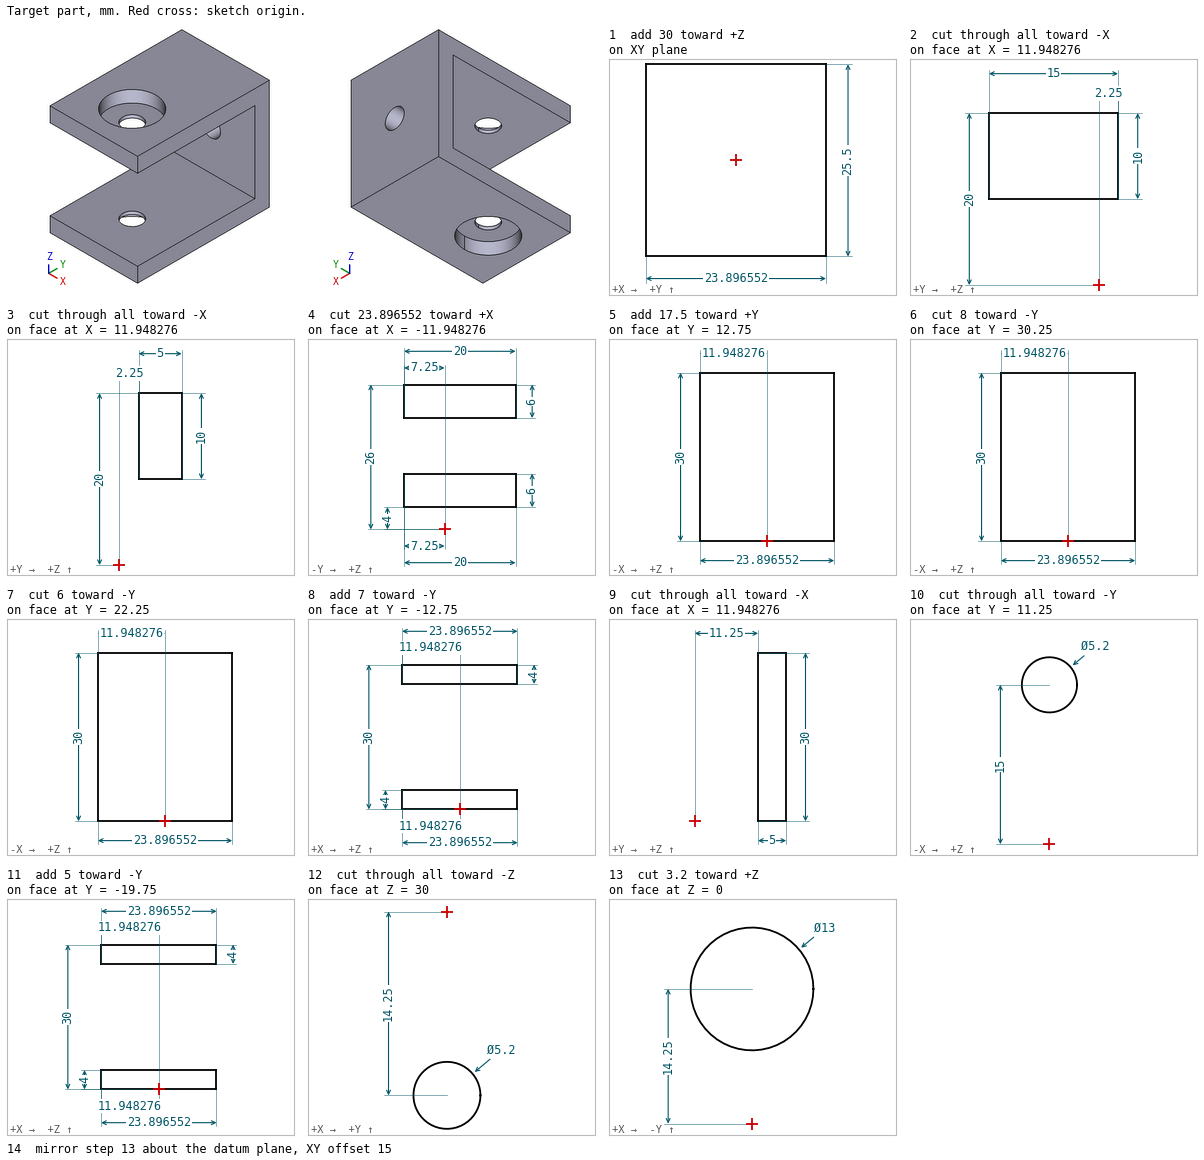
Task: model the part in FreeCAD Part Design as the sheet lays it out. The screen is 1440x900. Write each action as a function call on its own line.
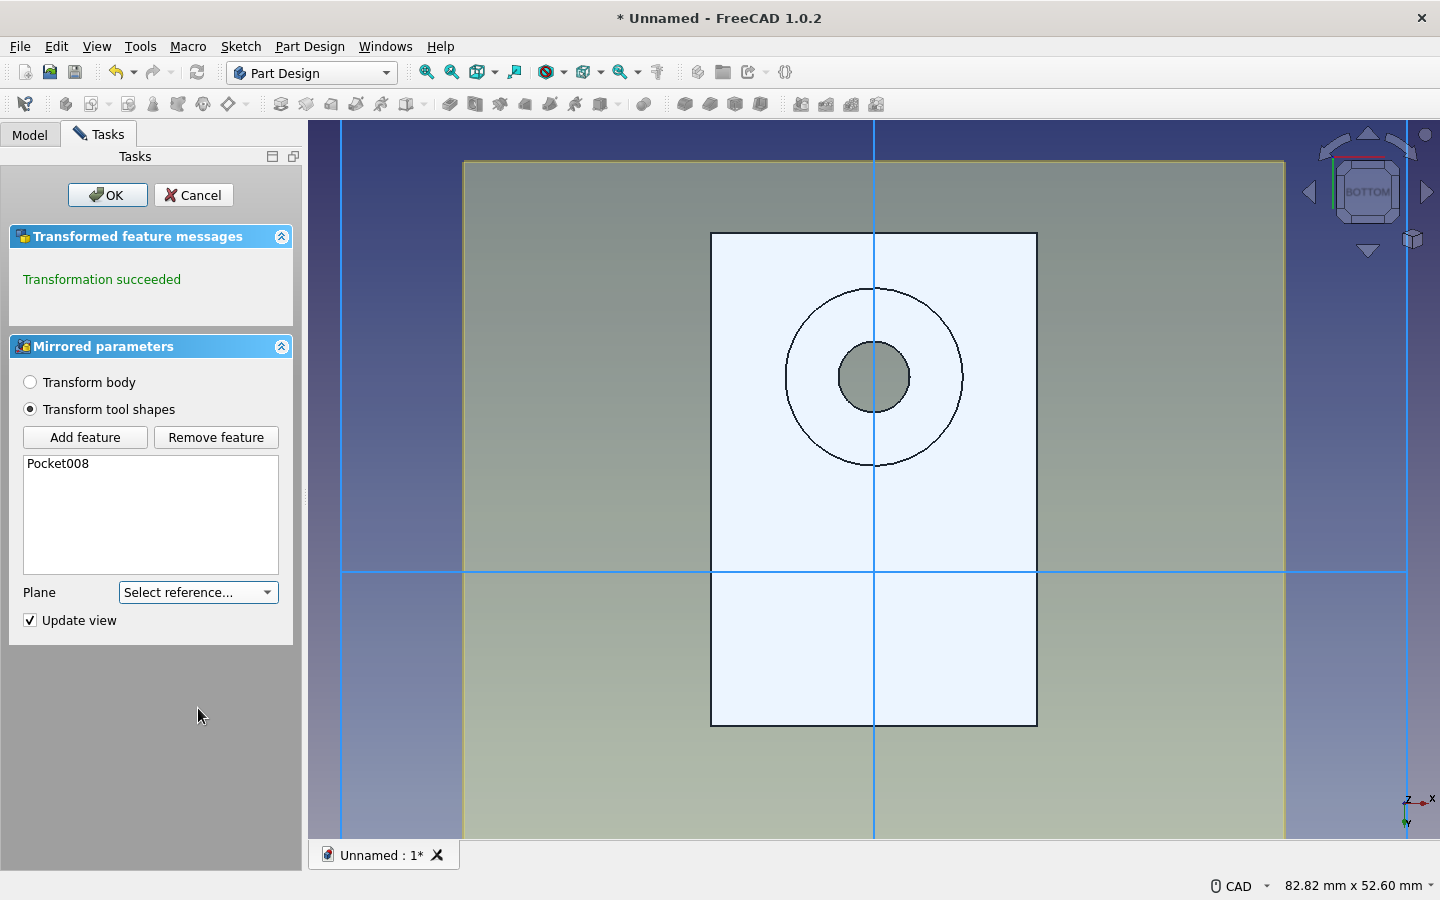
click(30, 134)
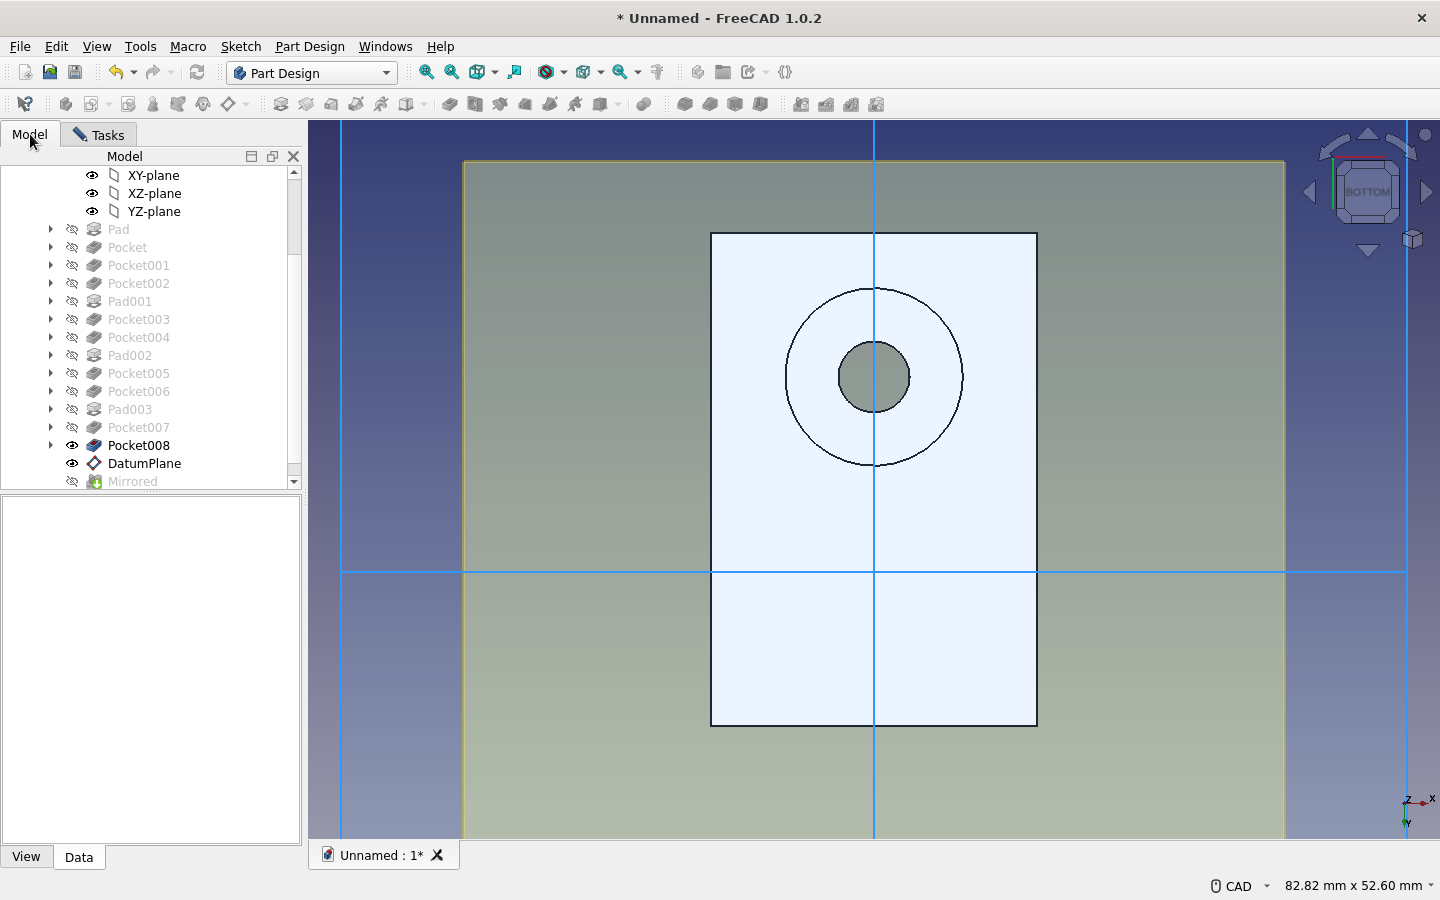
click(117, 463)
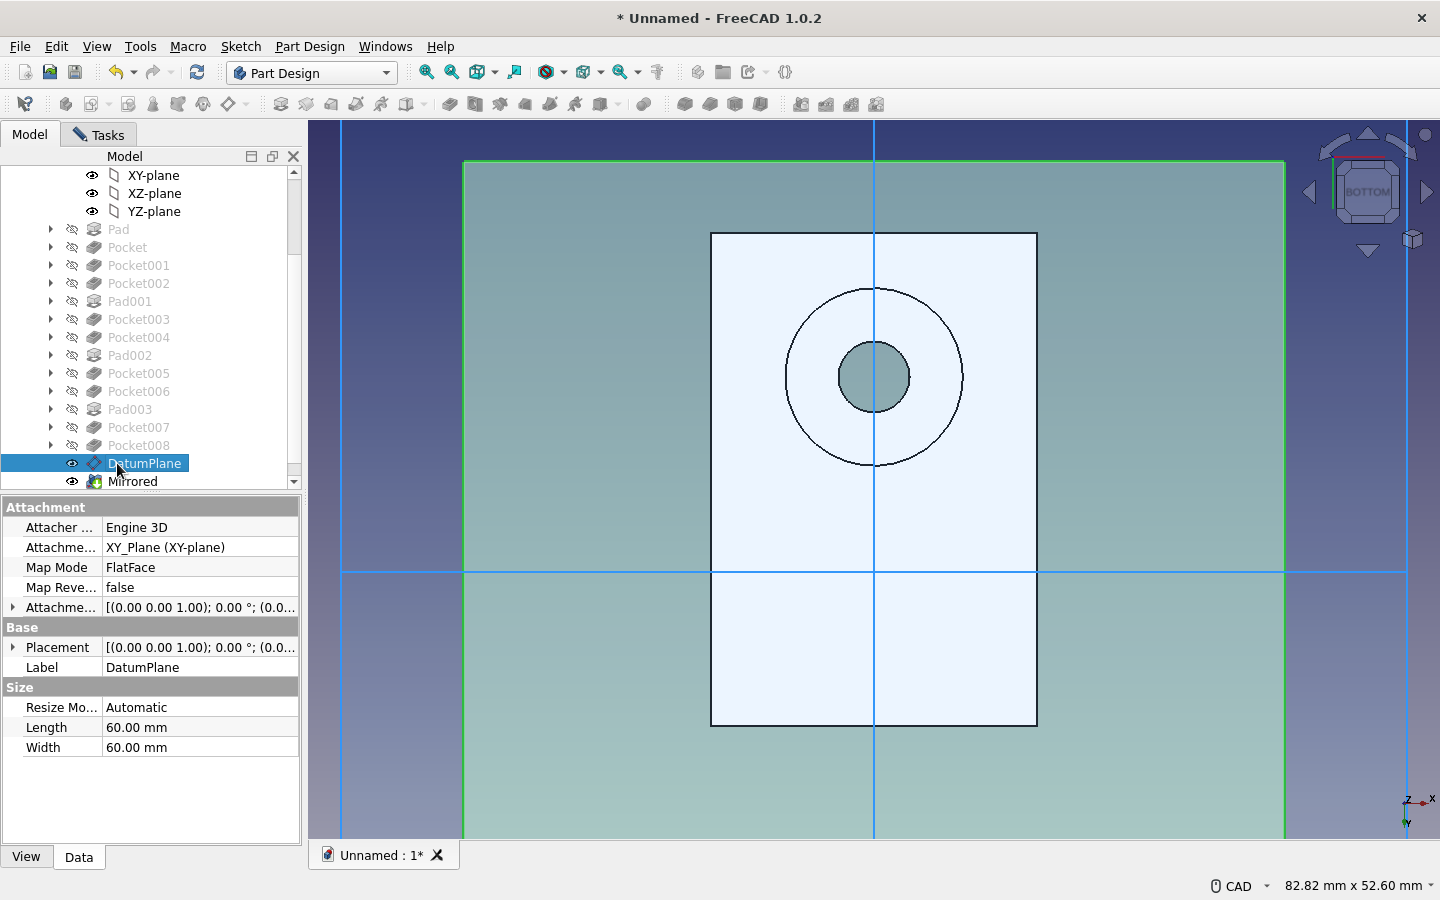
click(98, 134)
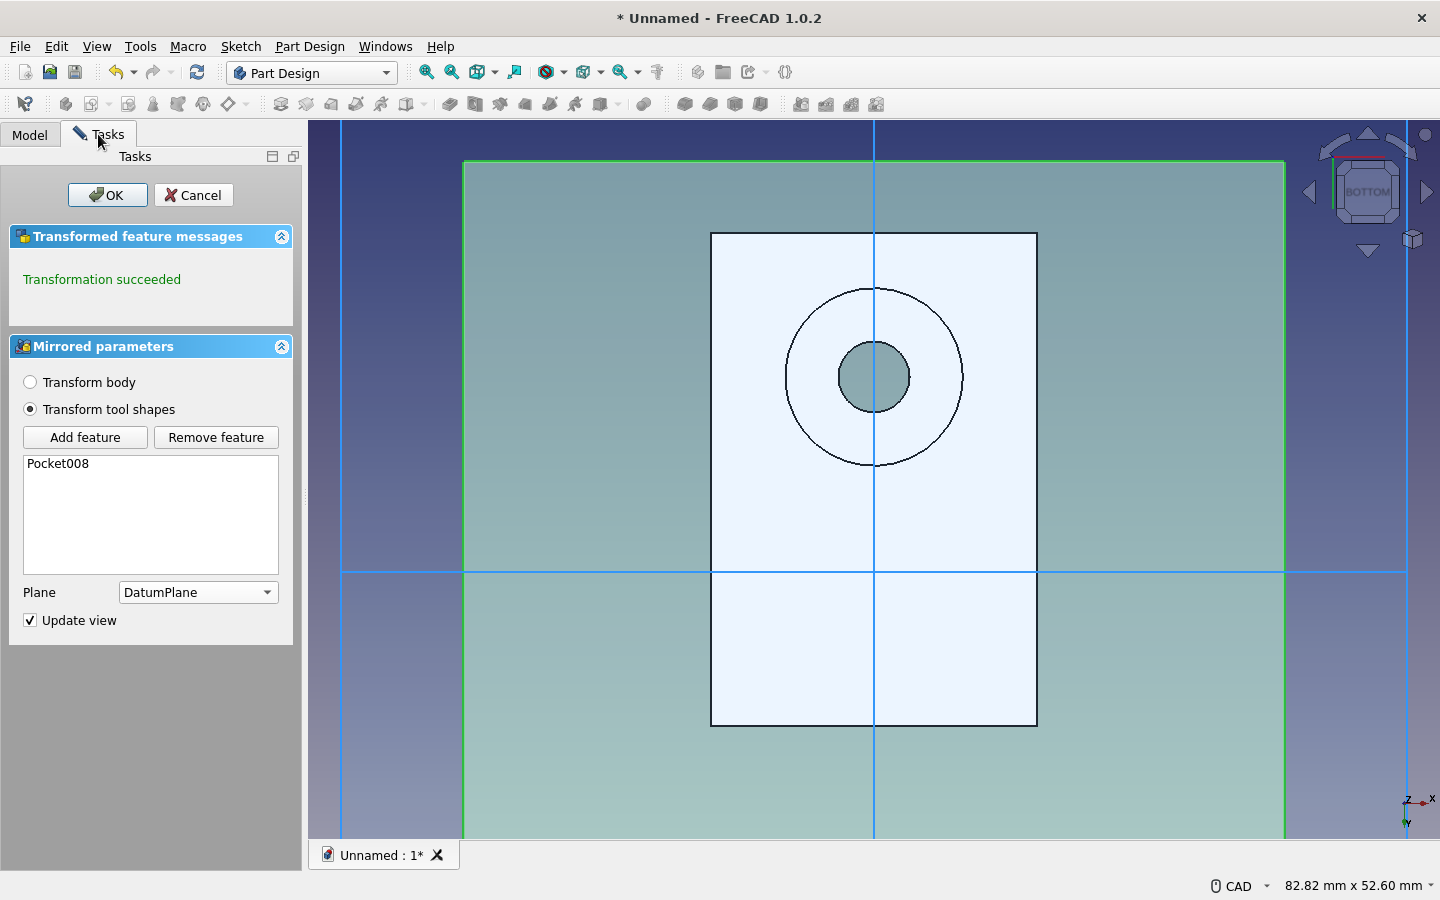
click(108, 195)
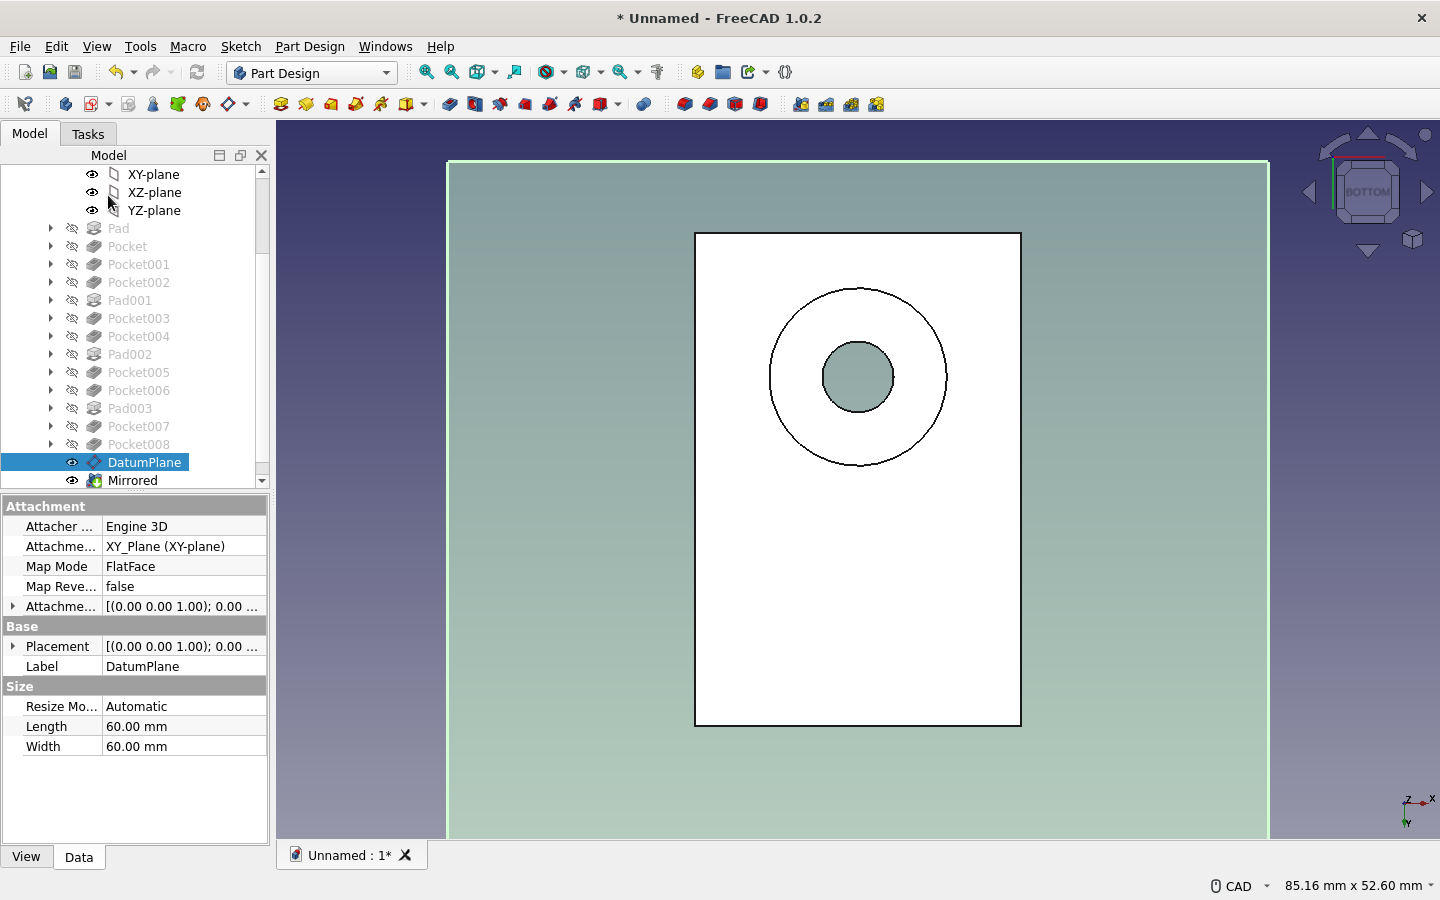
click(117, 462)
key(space)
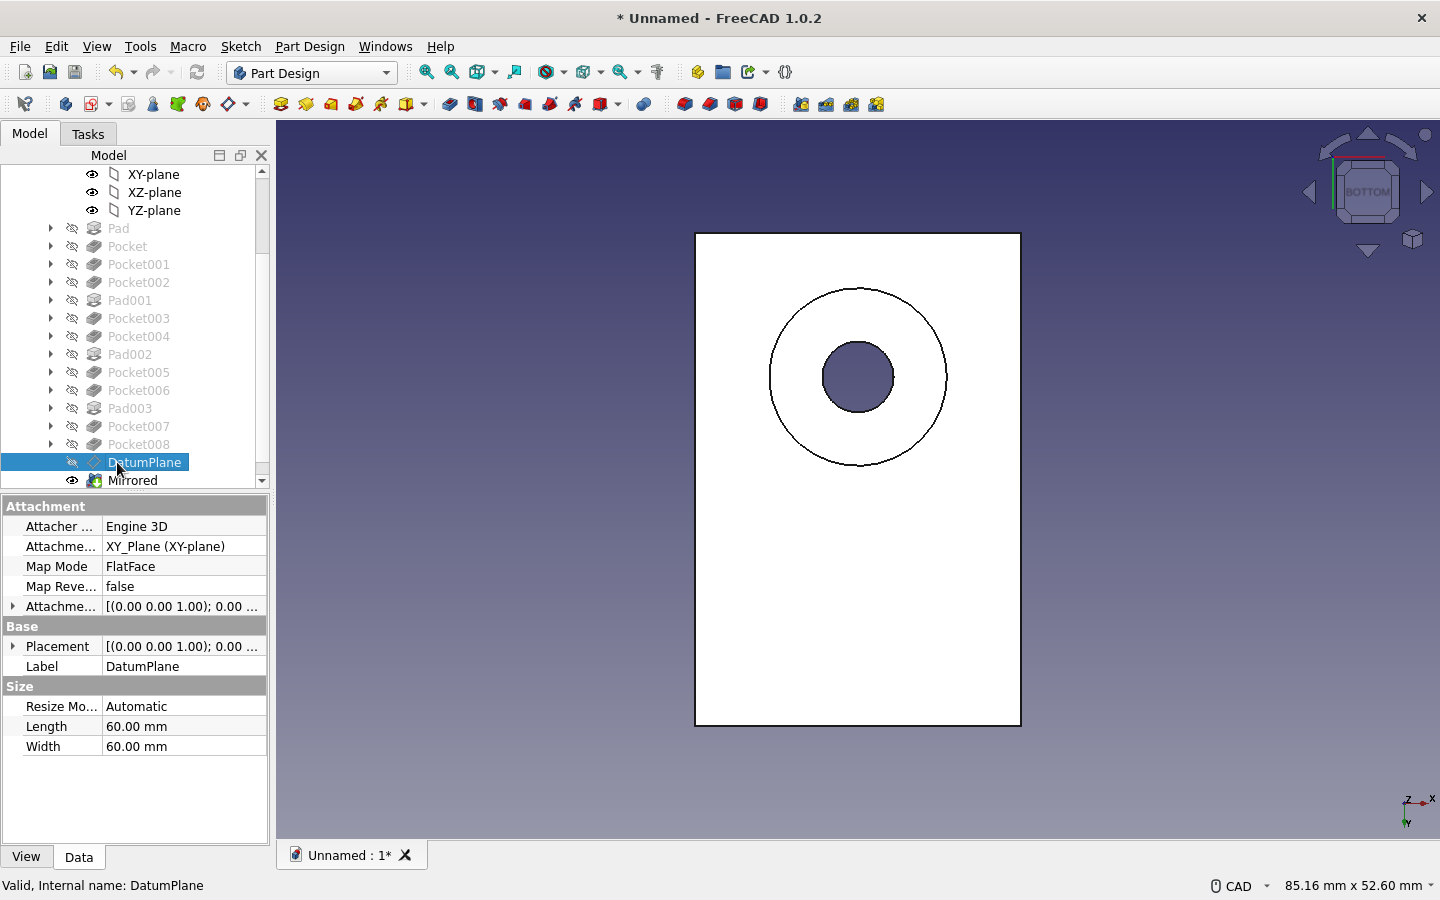
key(0)